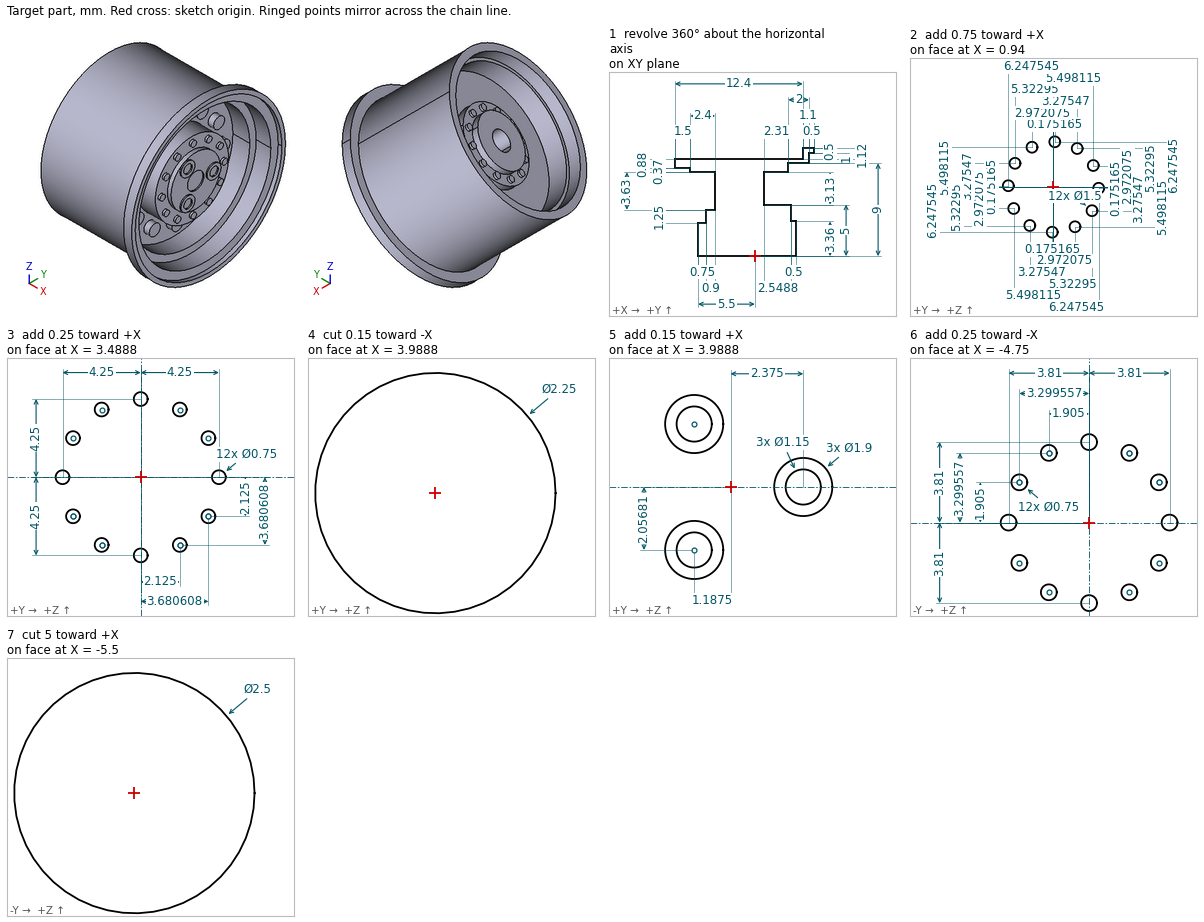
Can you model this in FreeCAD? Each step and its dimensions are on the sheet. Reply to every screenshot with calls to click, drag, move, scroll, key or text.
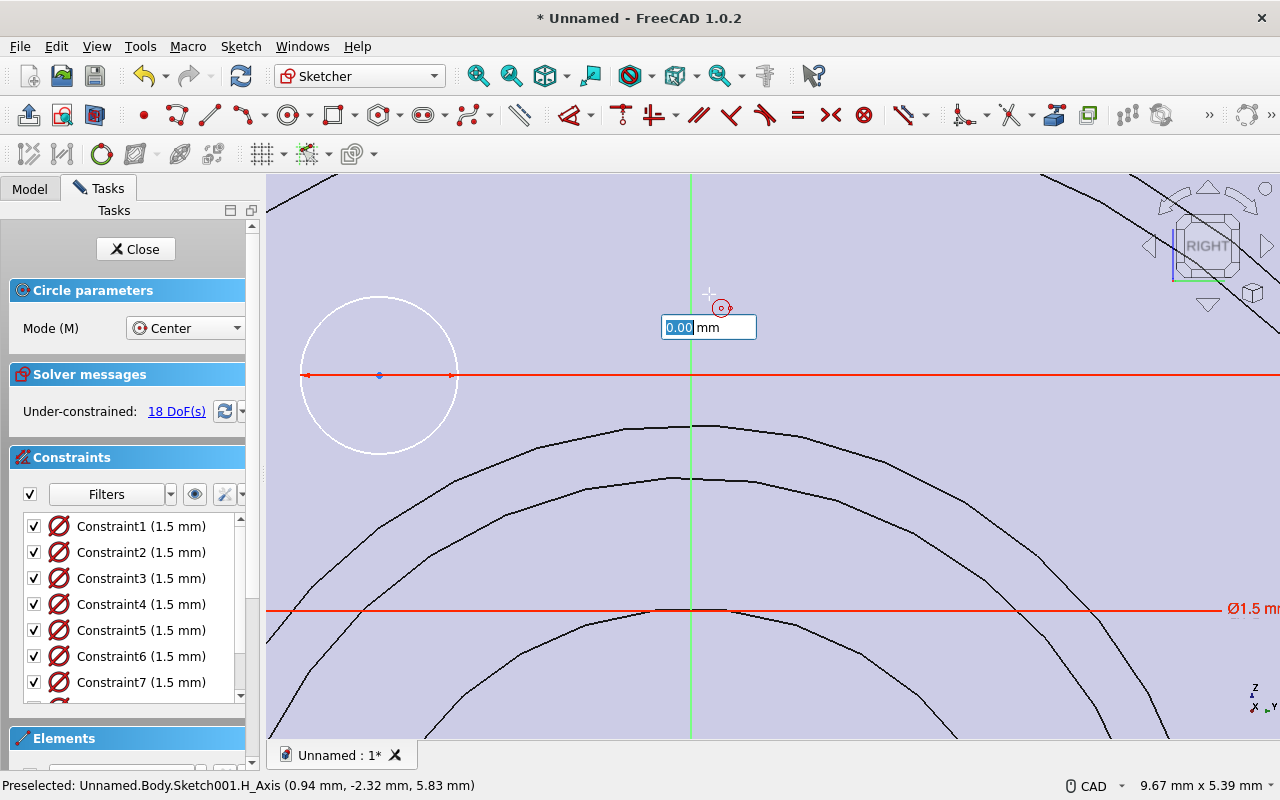
scroll(709, 295, down, 7)
move(723, 281)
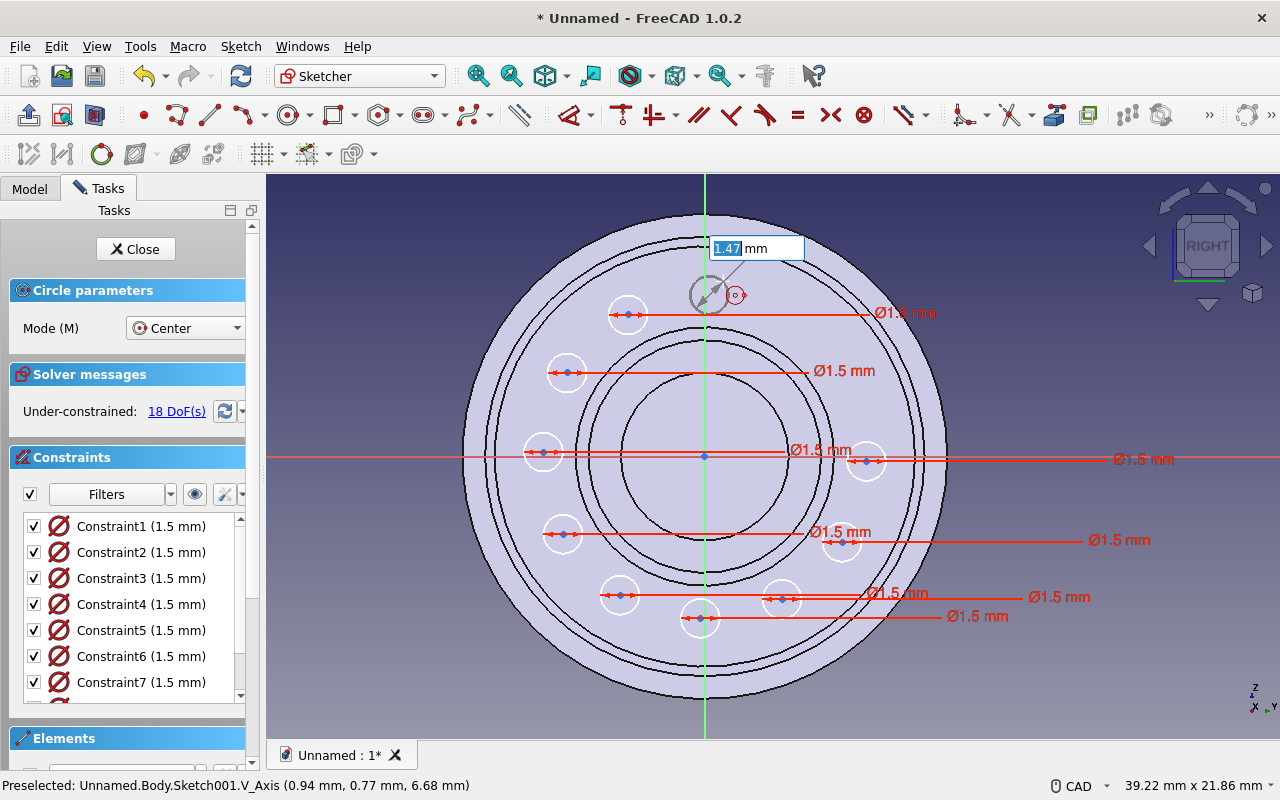
text(1.5)
key(Return)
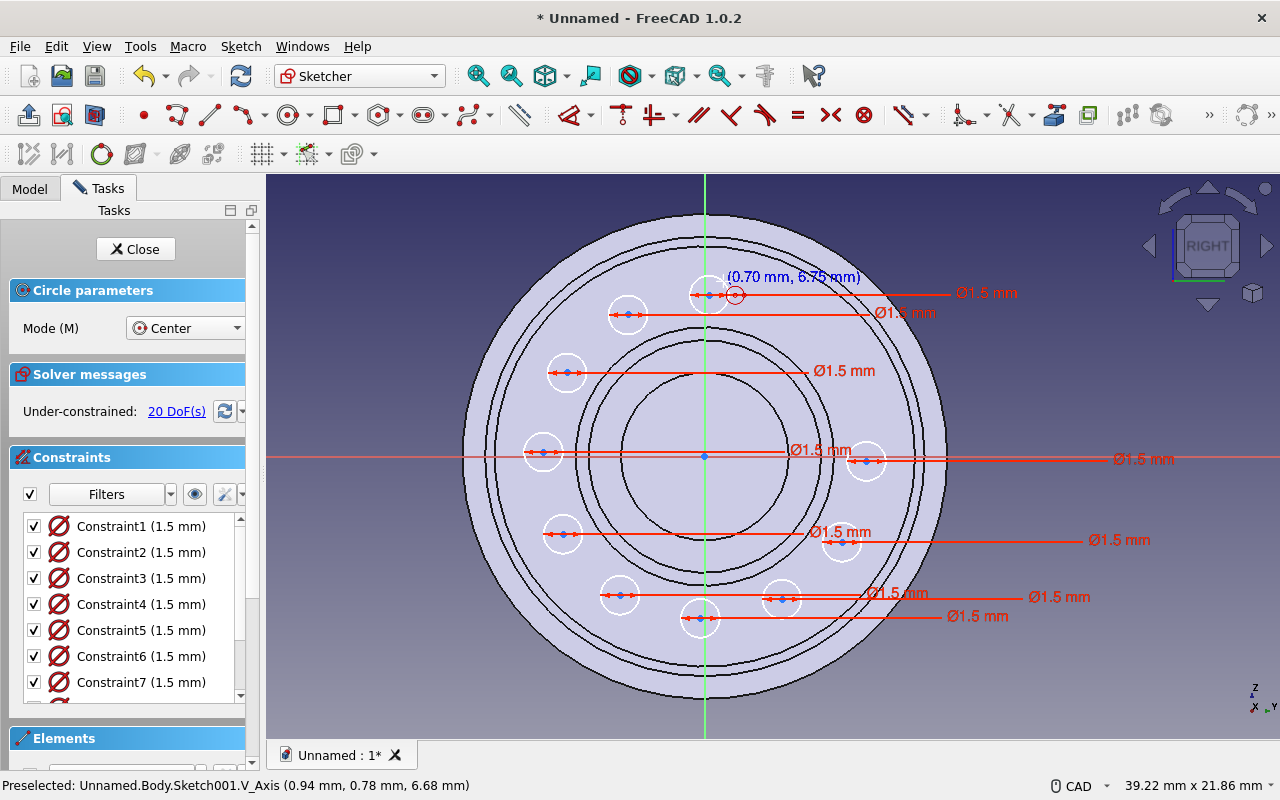
click(790, 319)
move(803, 305)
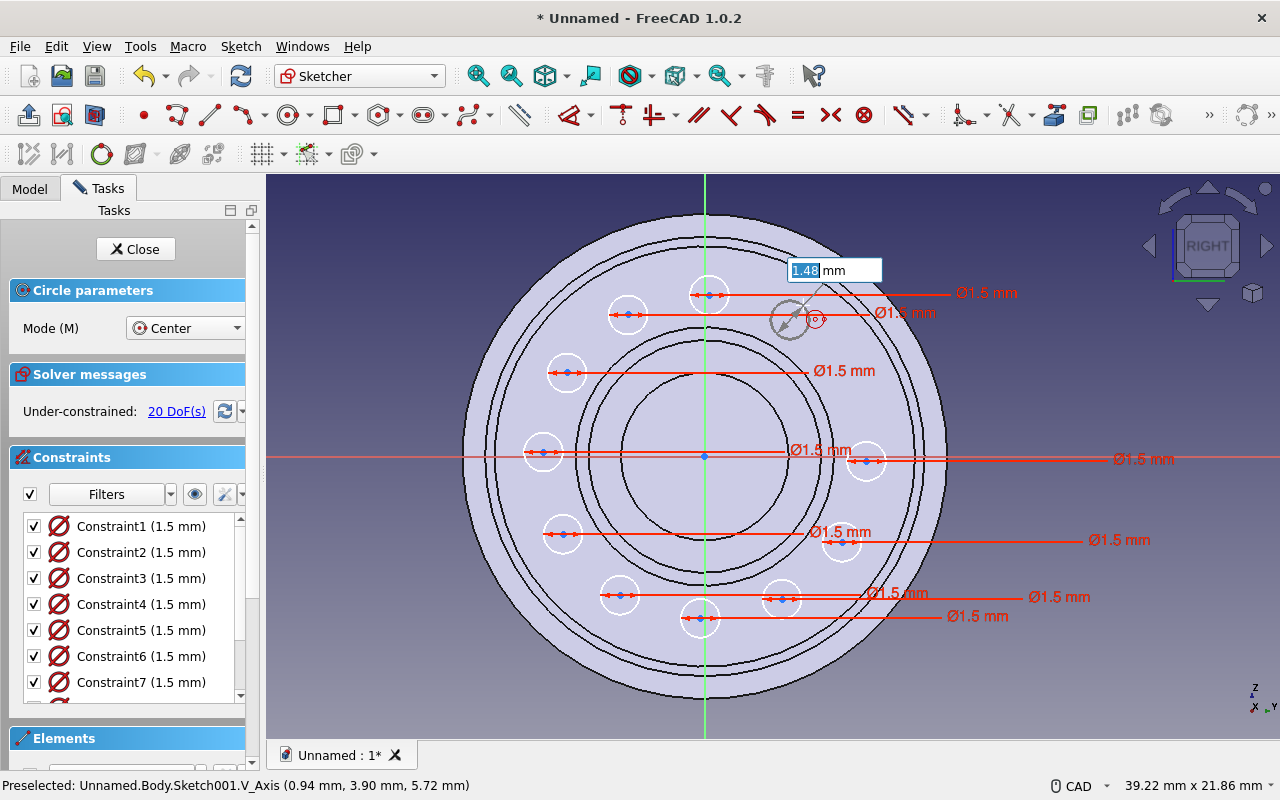
text(1.5)
key(Return)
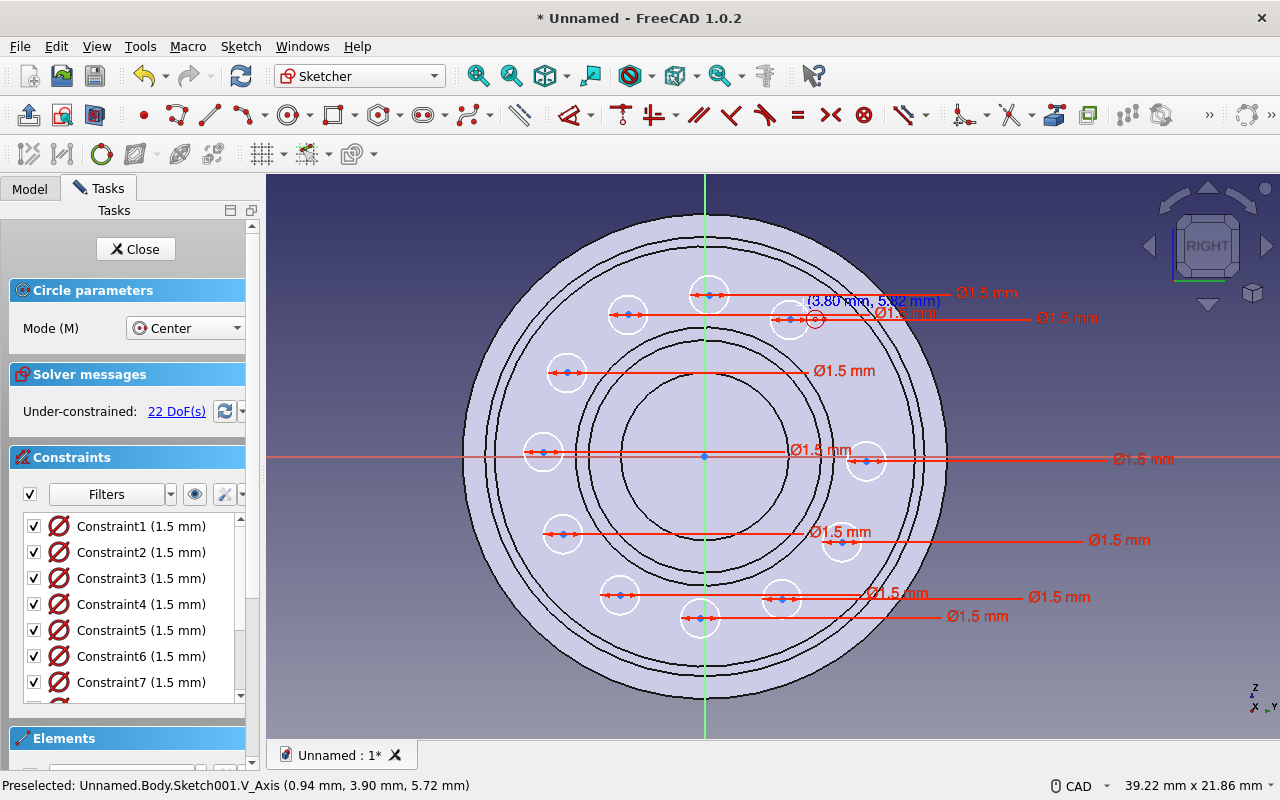
click(847, 380)
move(861, 366)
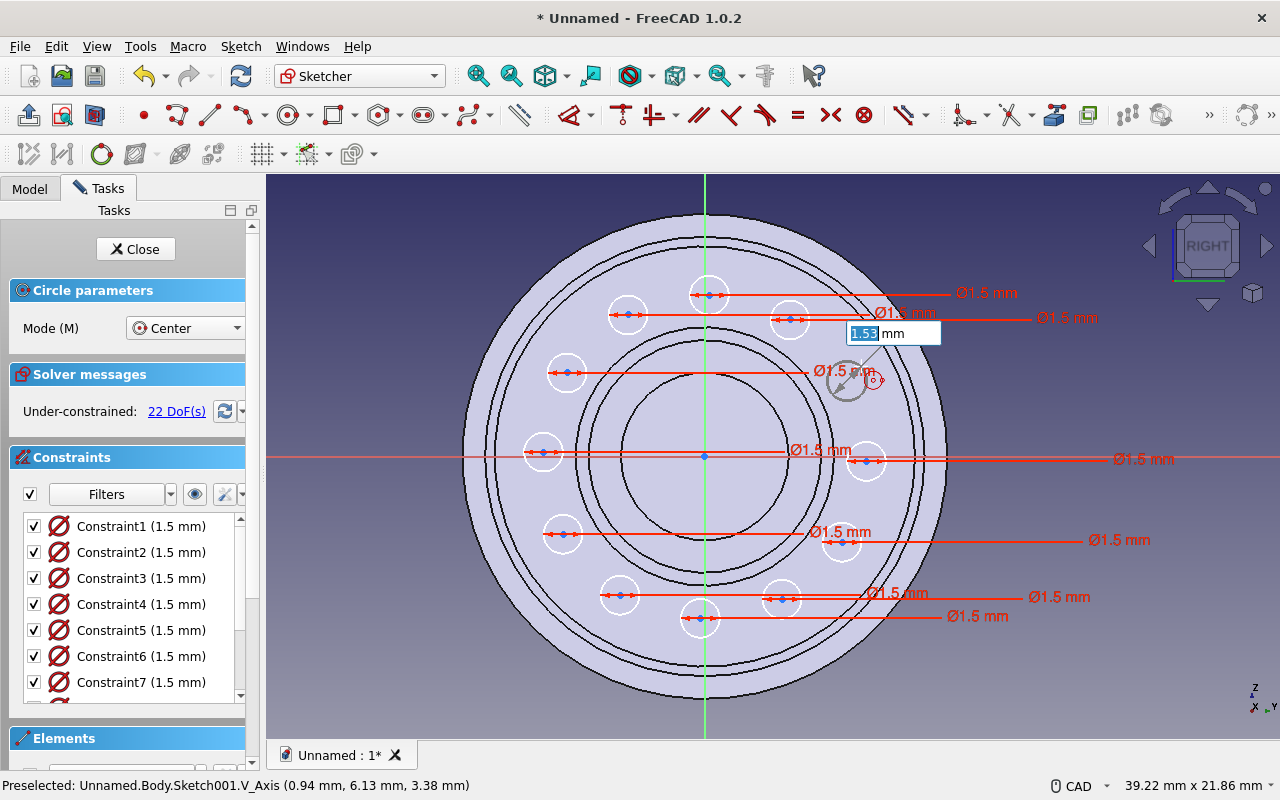
text(1.5)
key(Return)
key(Escape)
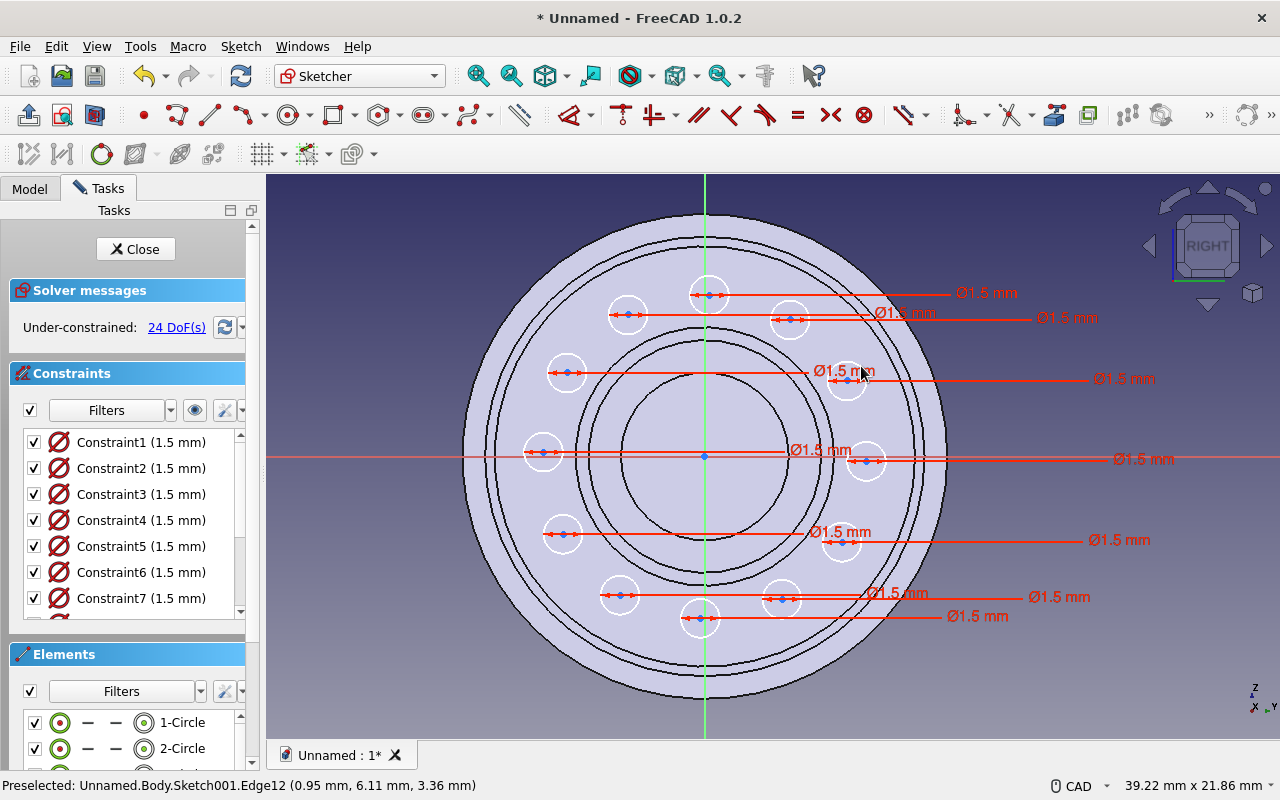
click(568, 116)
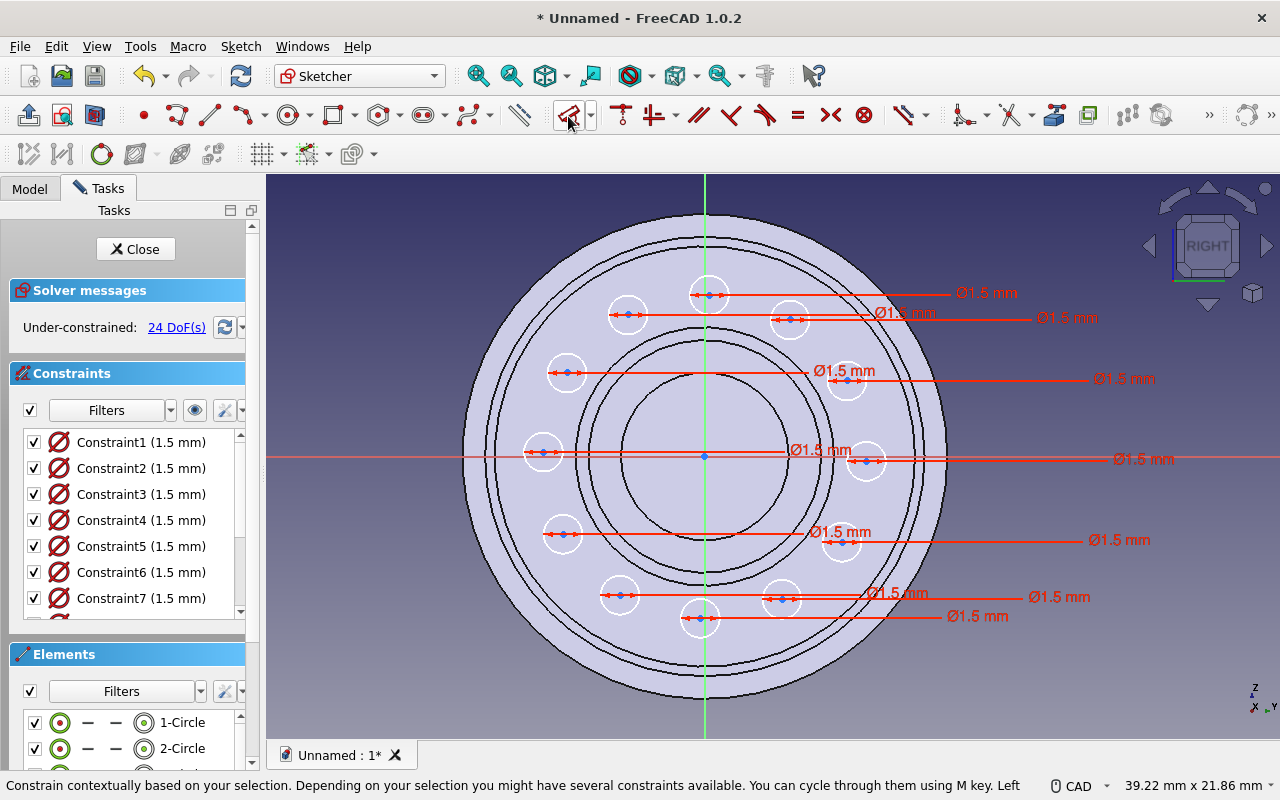
click(842, 542)
click(742, 576)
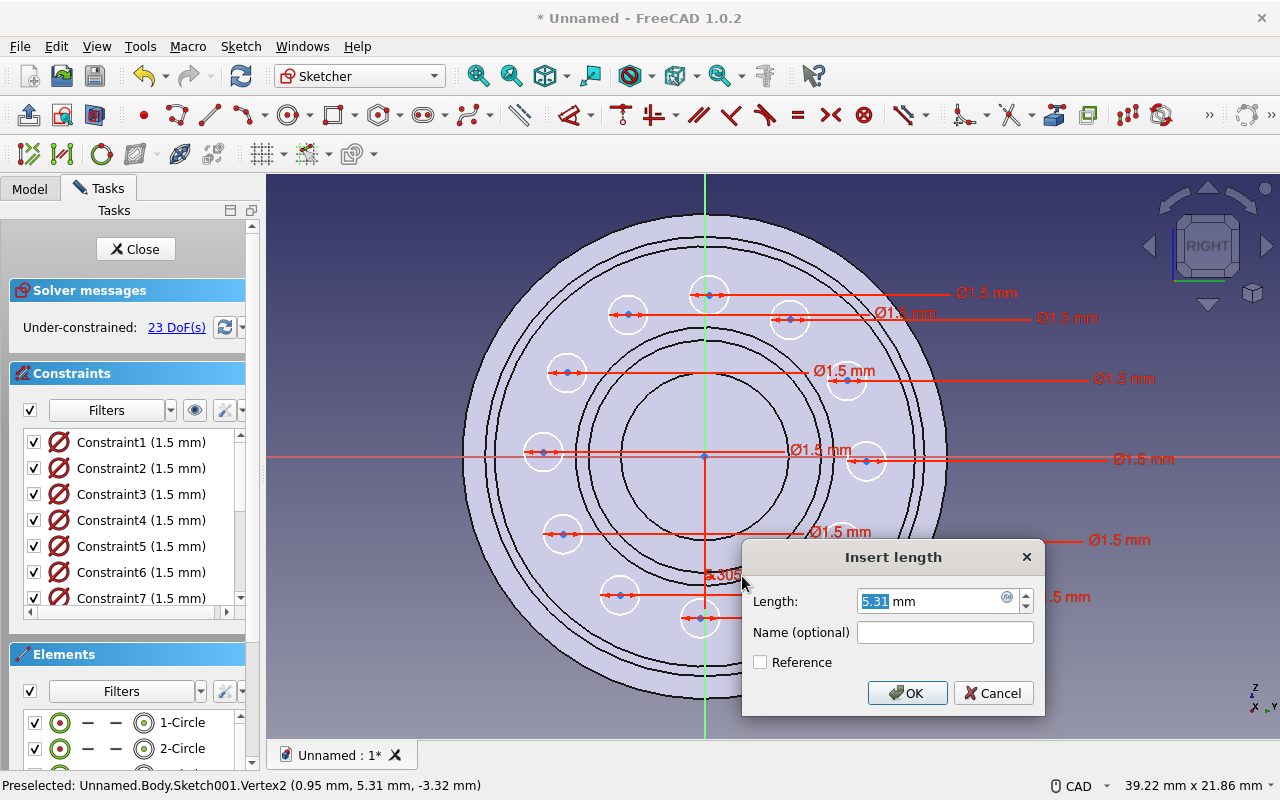
text(5.32295)
key(Return)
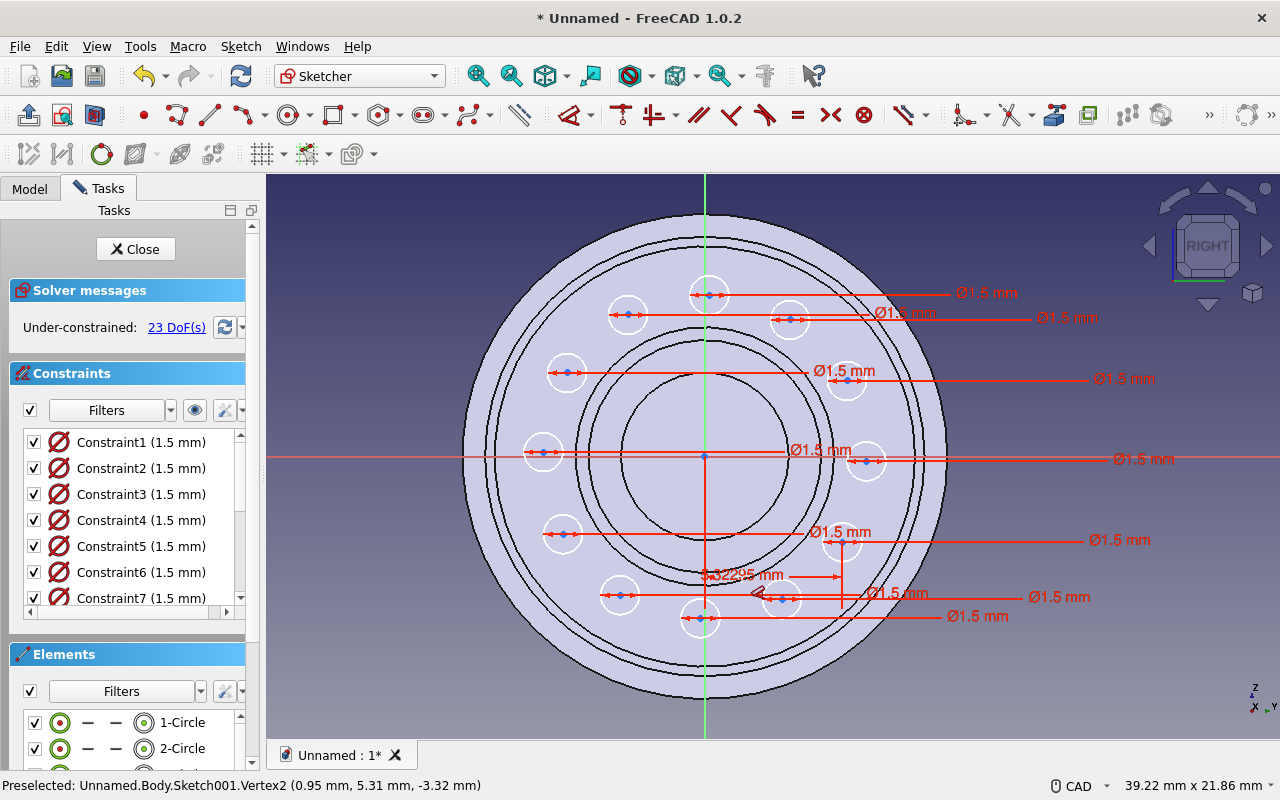
click(842, 542)
click(876, 499)